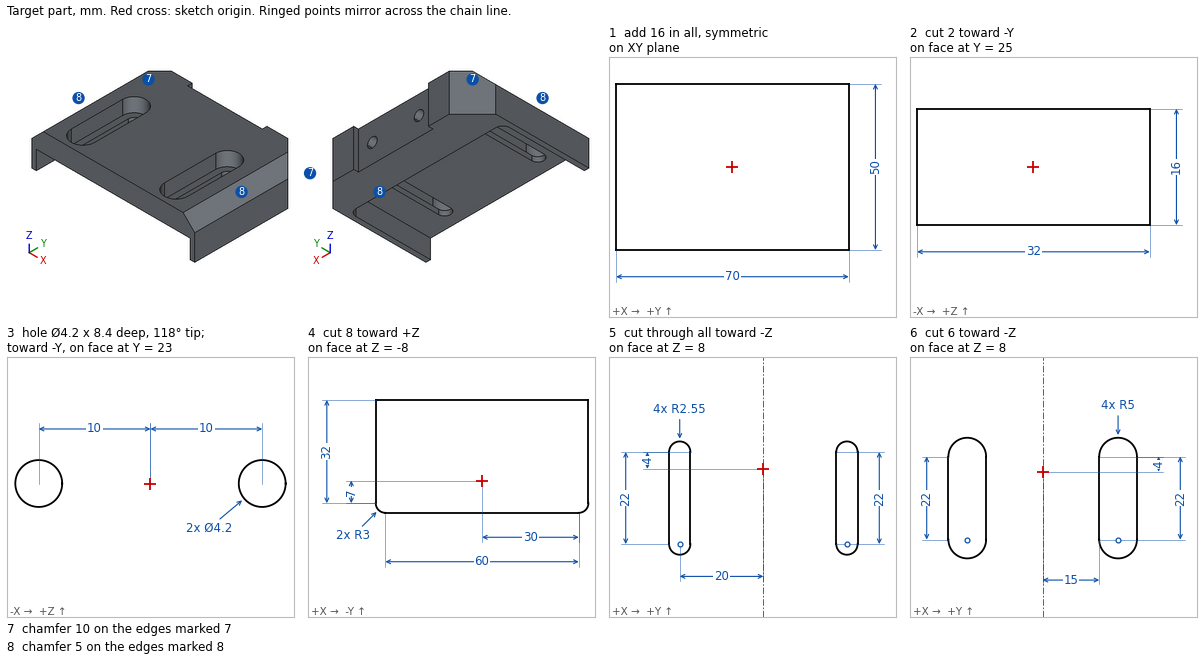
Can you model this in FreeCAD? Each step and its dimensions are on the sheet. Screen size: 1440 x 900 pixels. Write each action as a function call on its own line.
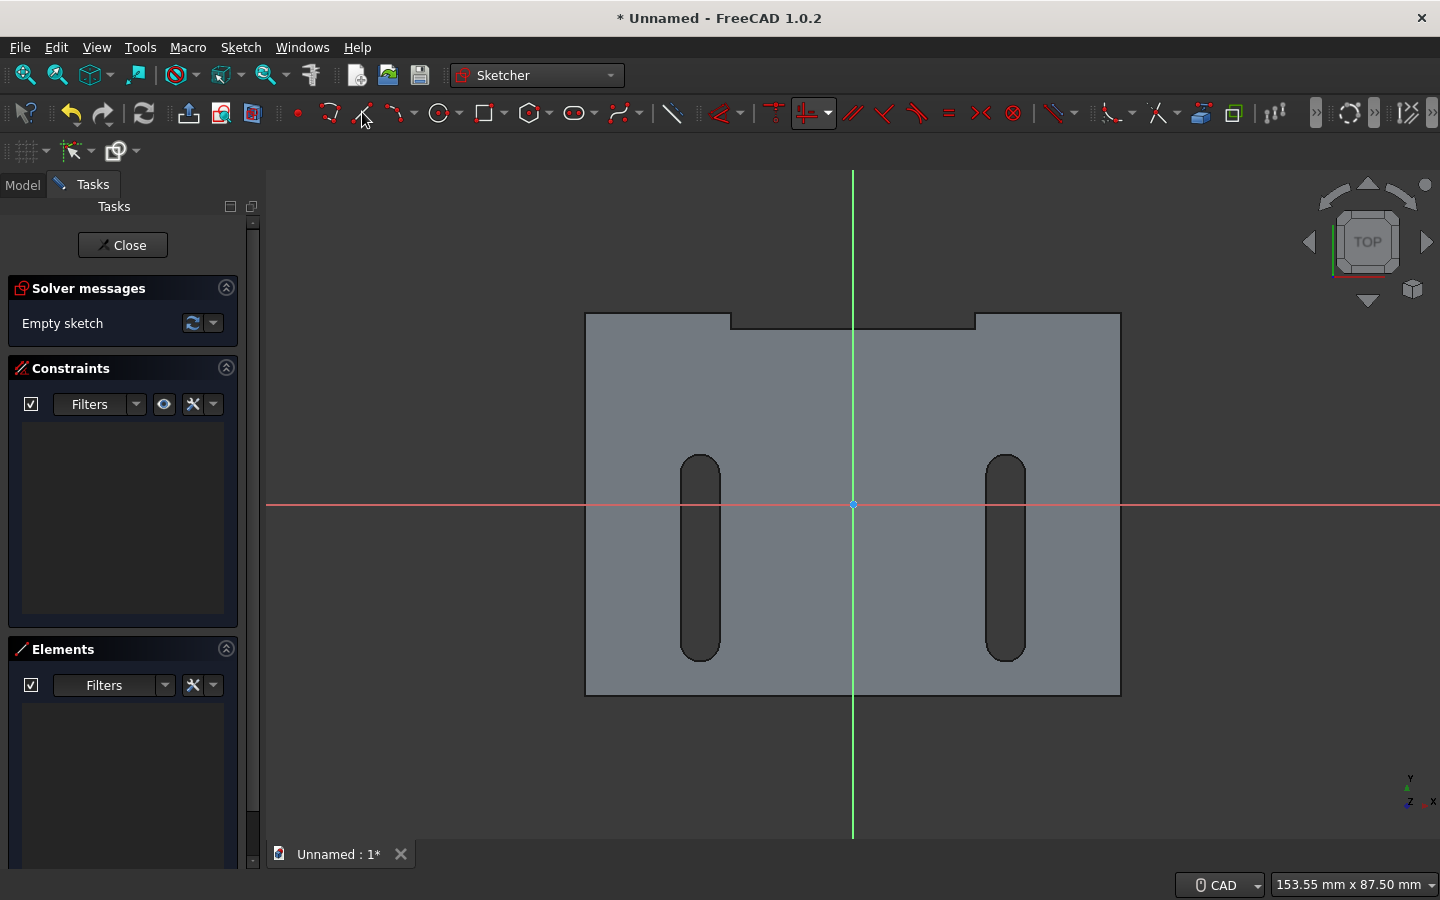
scroll(936, 623, up, 3)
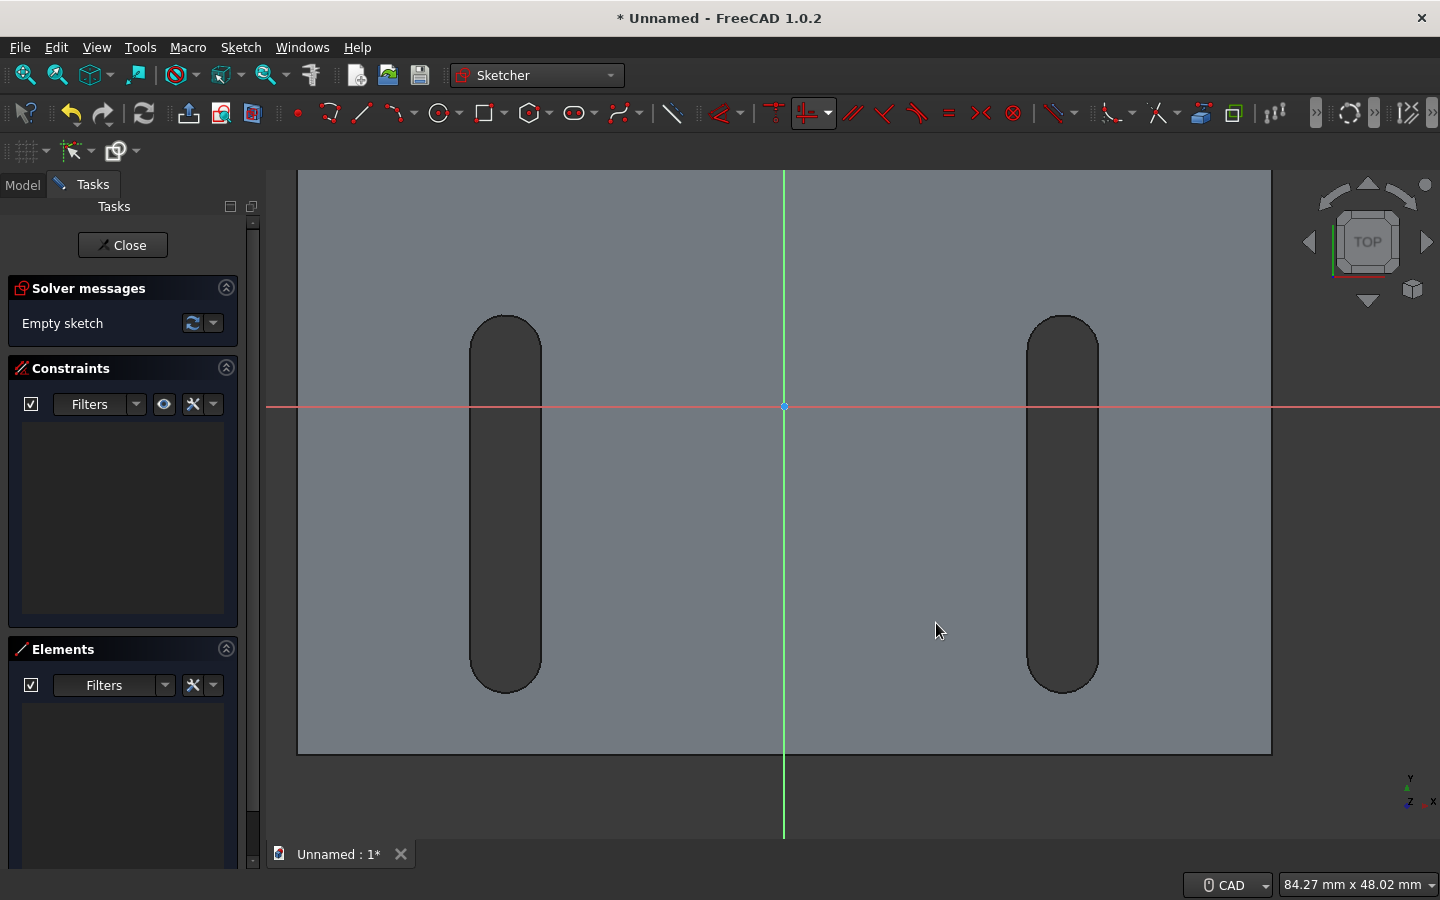
click(574, 114)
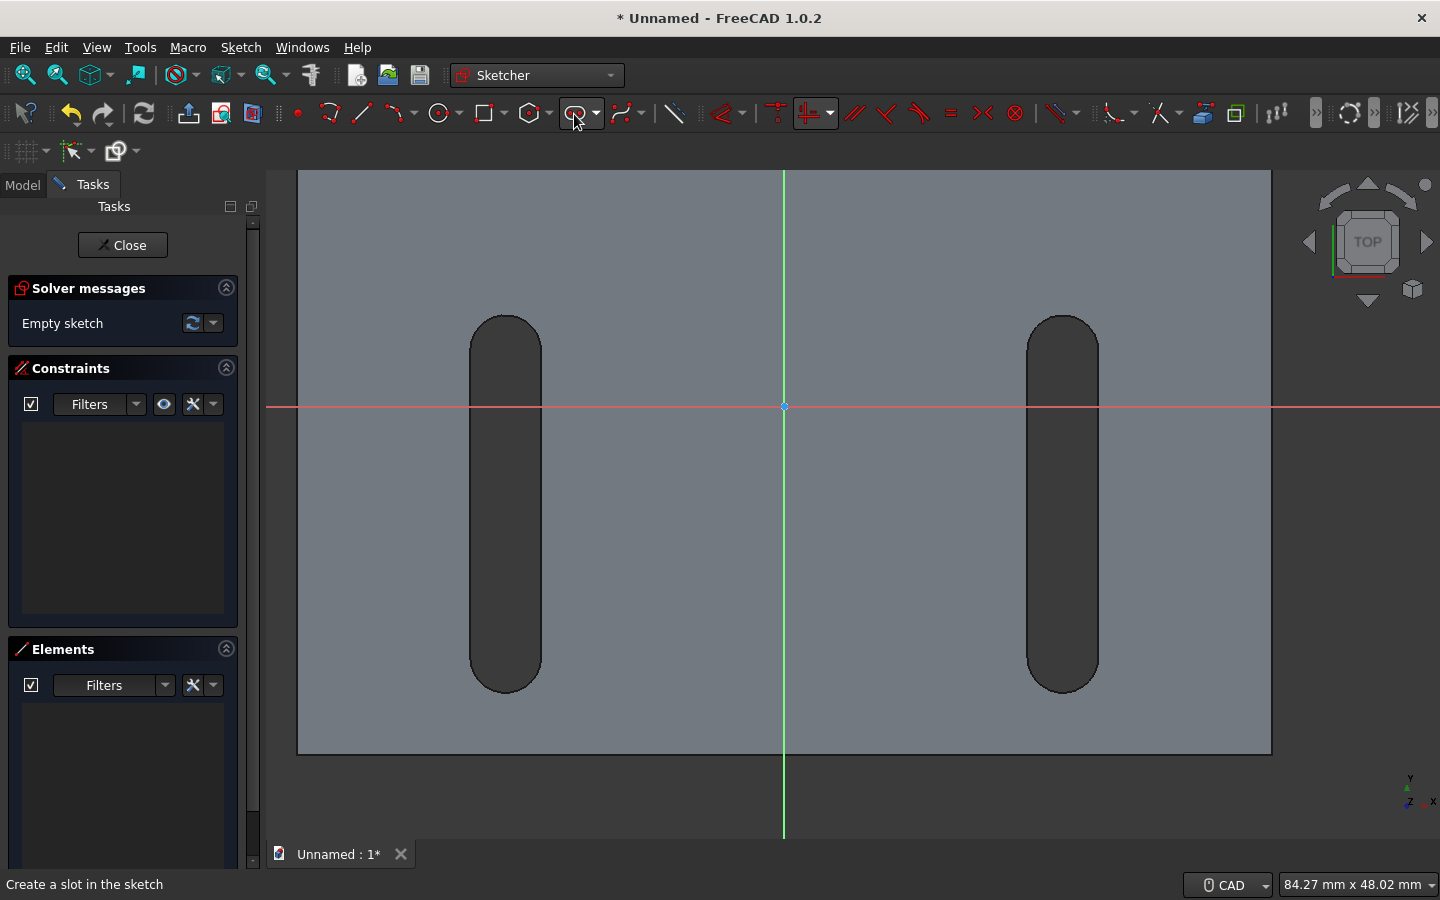
click(1063, 657)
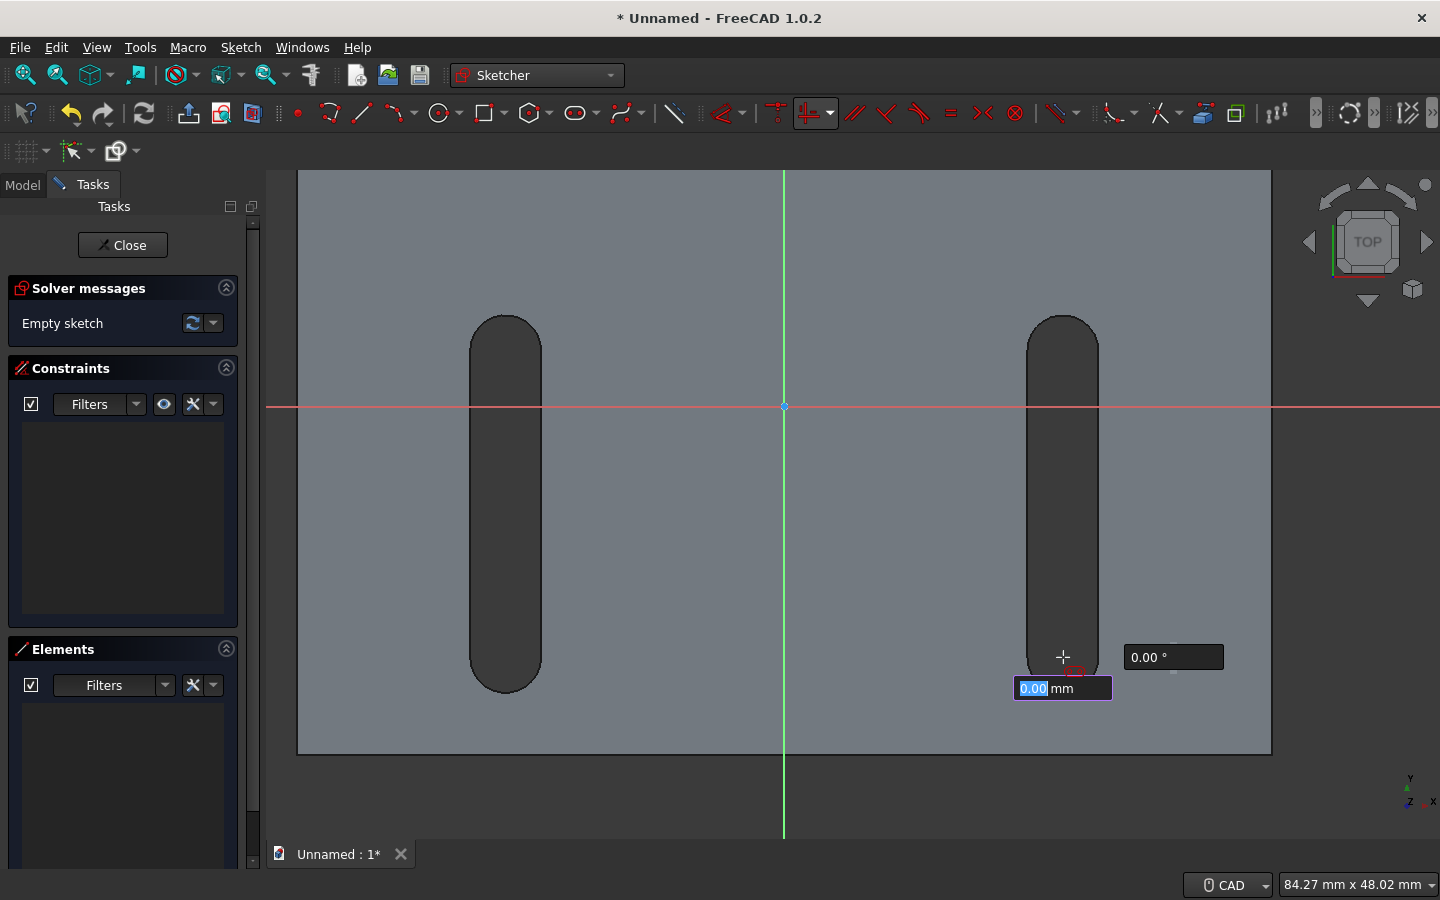
click(1063, 351)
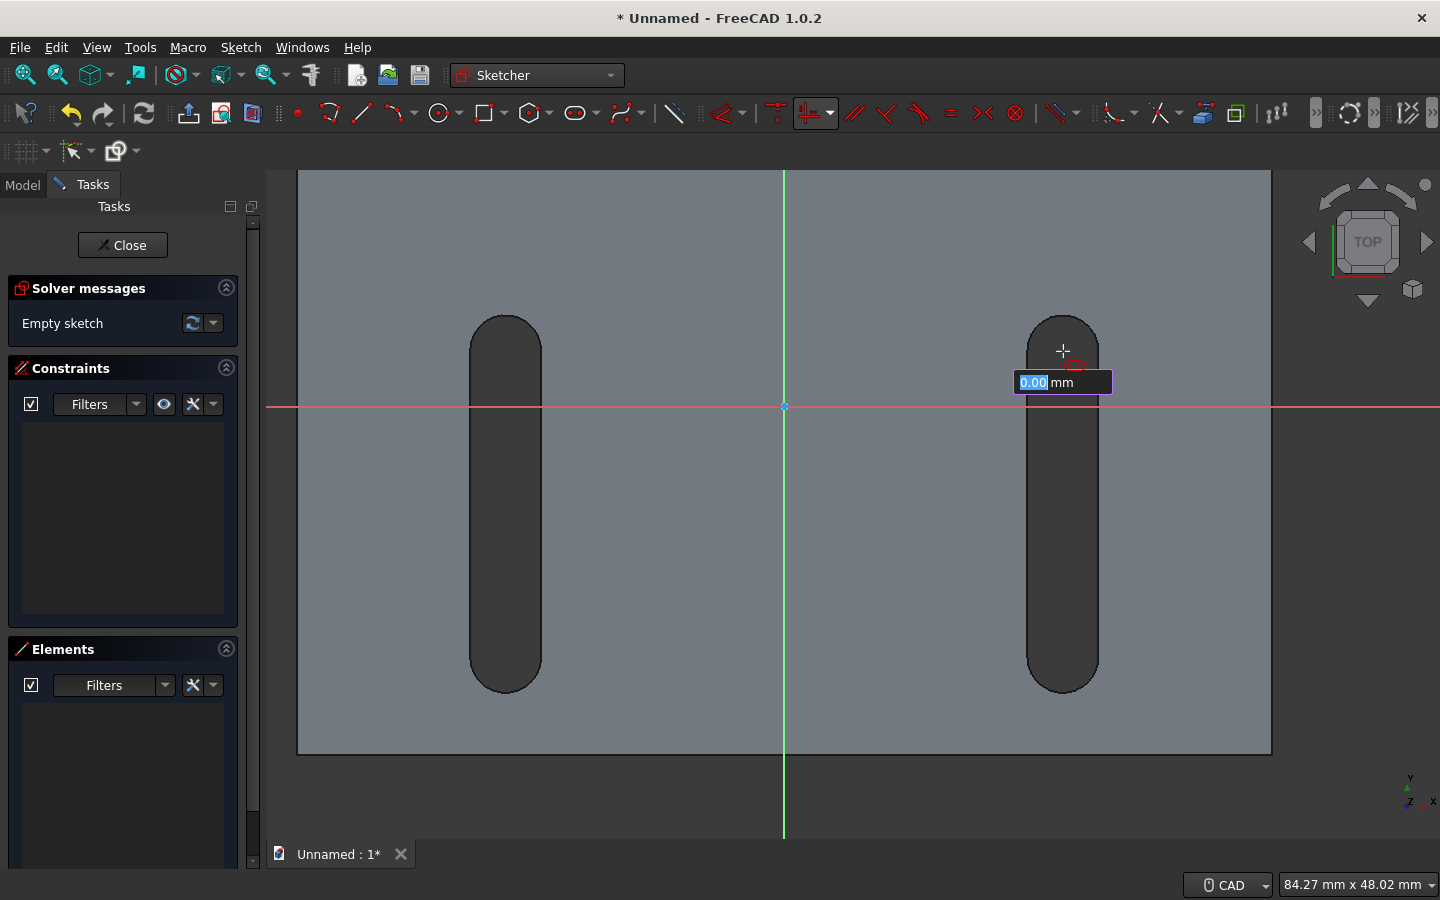
click(993, 504)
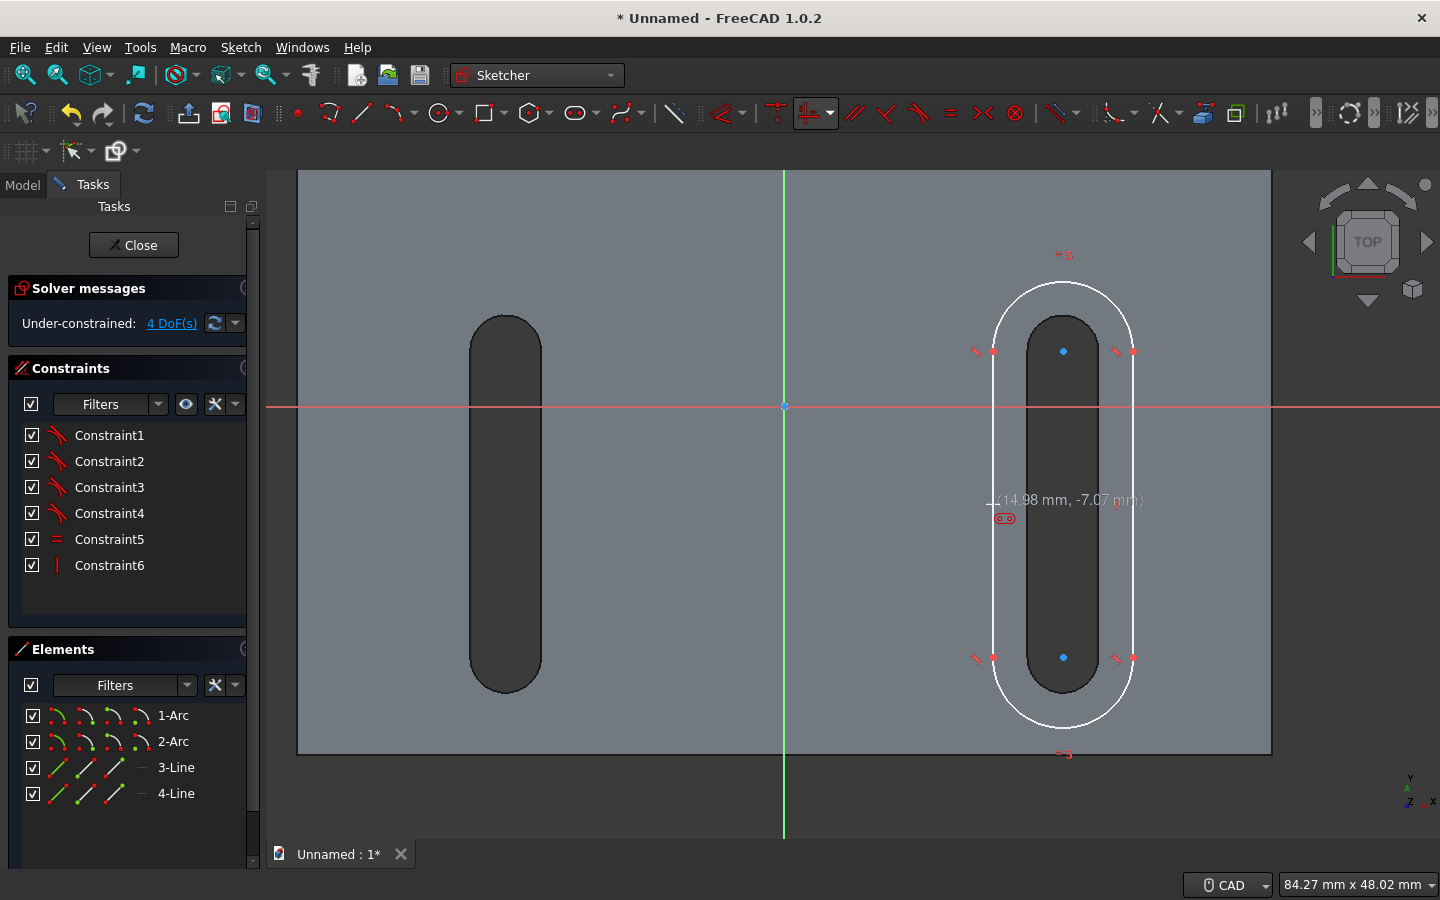
click(506, 657)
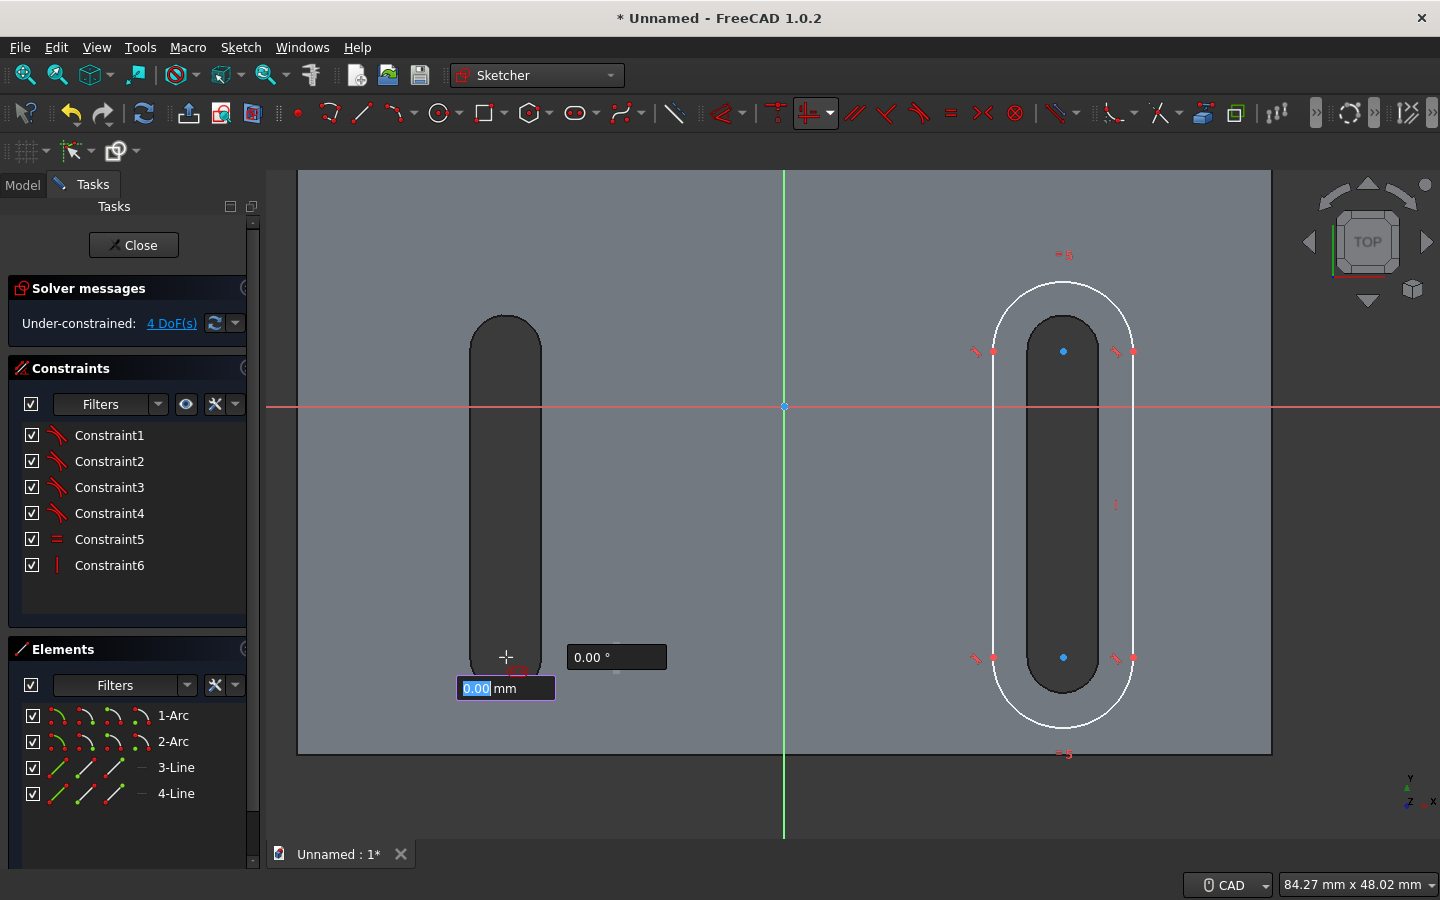
click(506, 351)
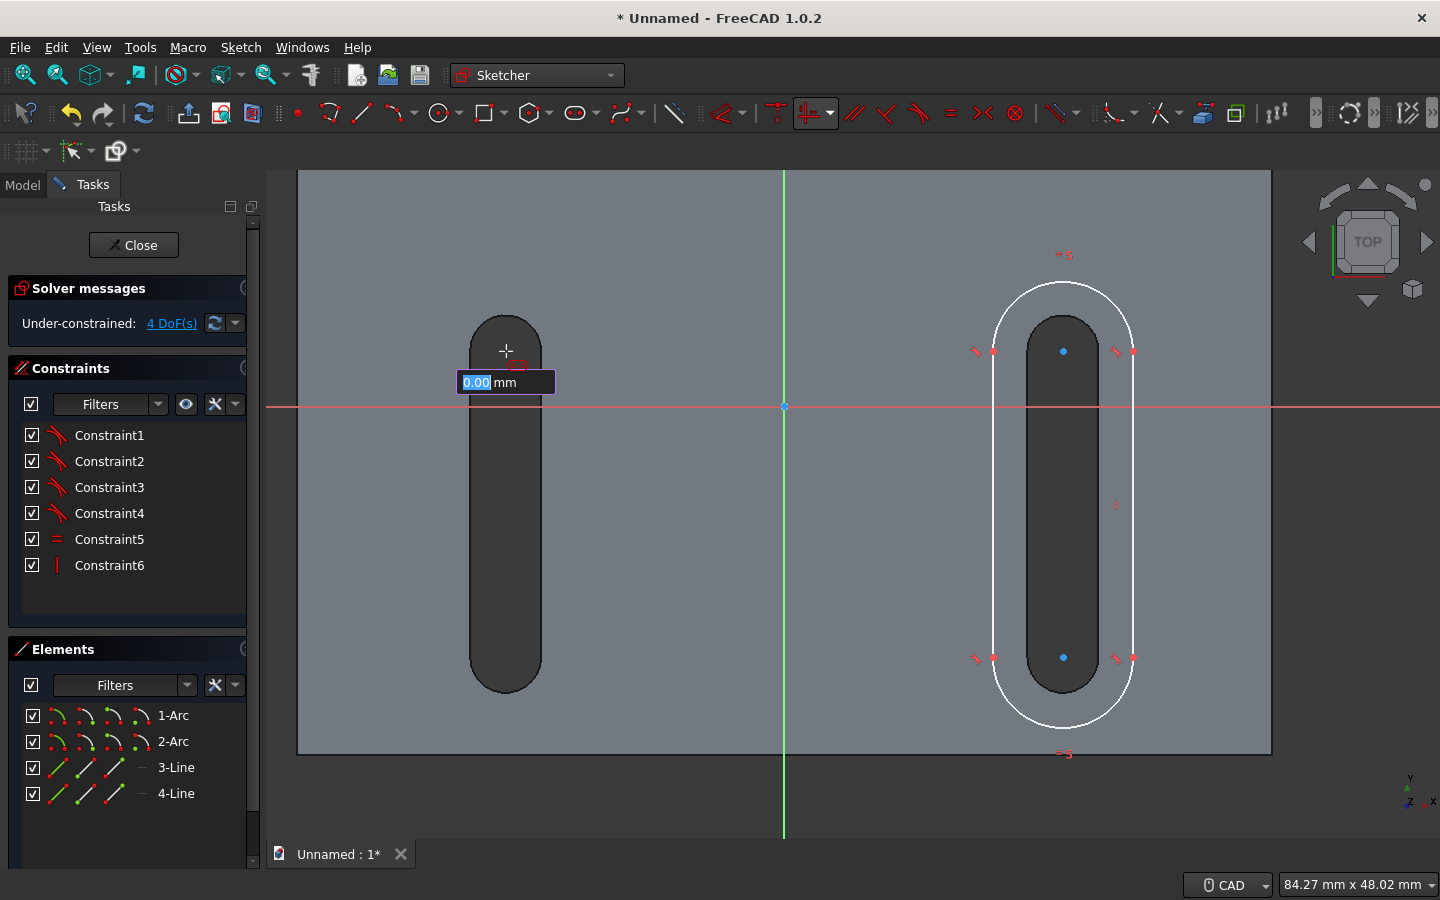
click(575, 504)
key(Escape)